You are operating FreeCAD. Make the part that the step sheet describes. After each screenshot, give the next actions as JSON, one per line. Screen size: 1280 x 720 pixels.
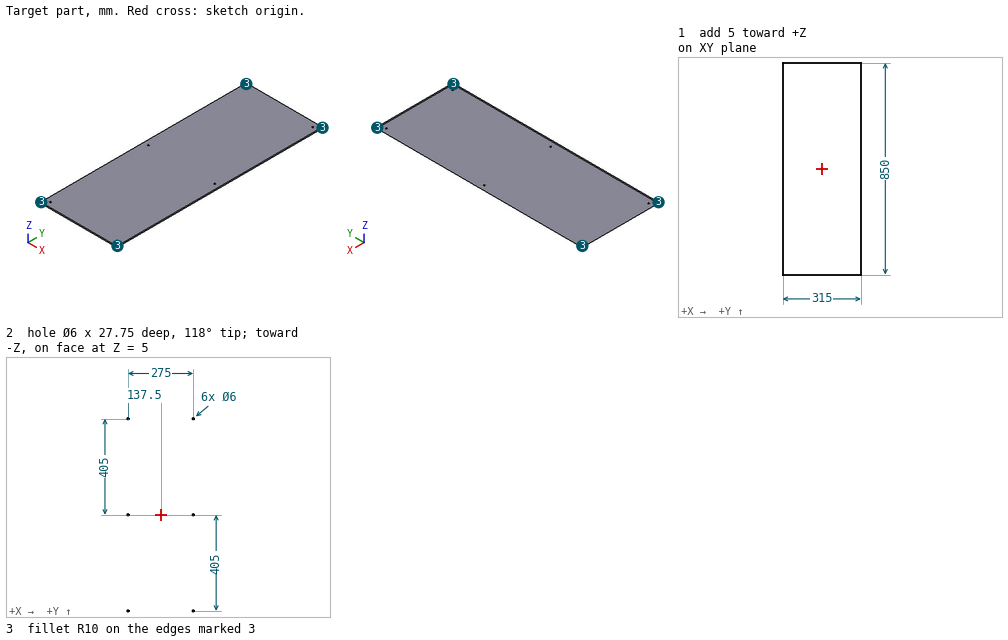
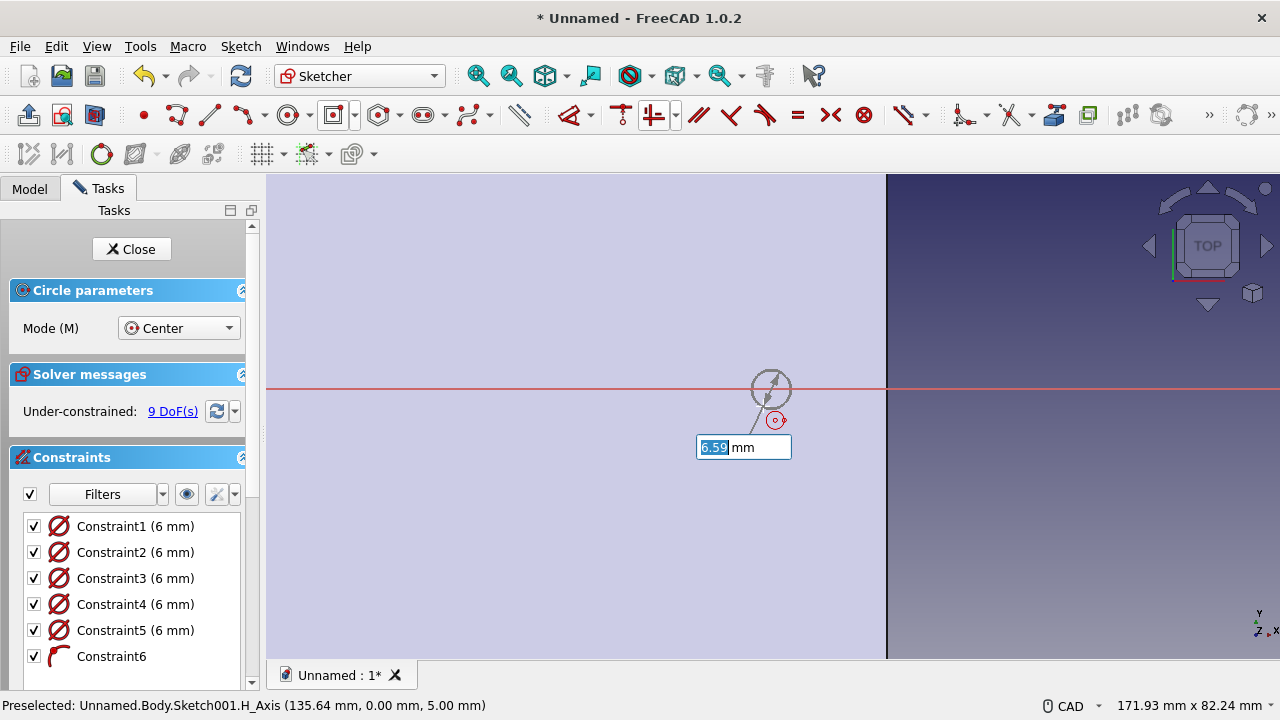
{"action": "type", "text": "6"}
{"action": "key", "text": "Return"}
{"action": "key", "text": "Escape"}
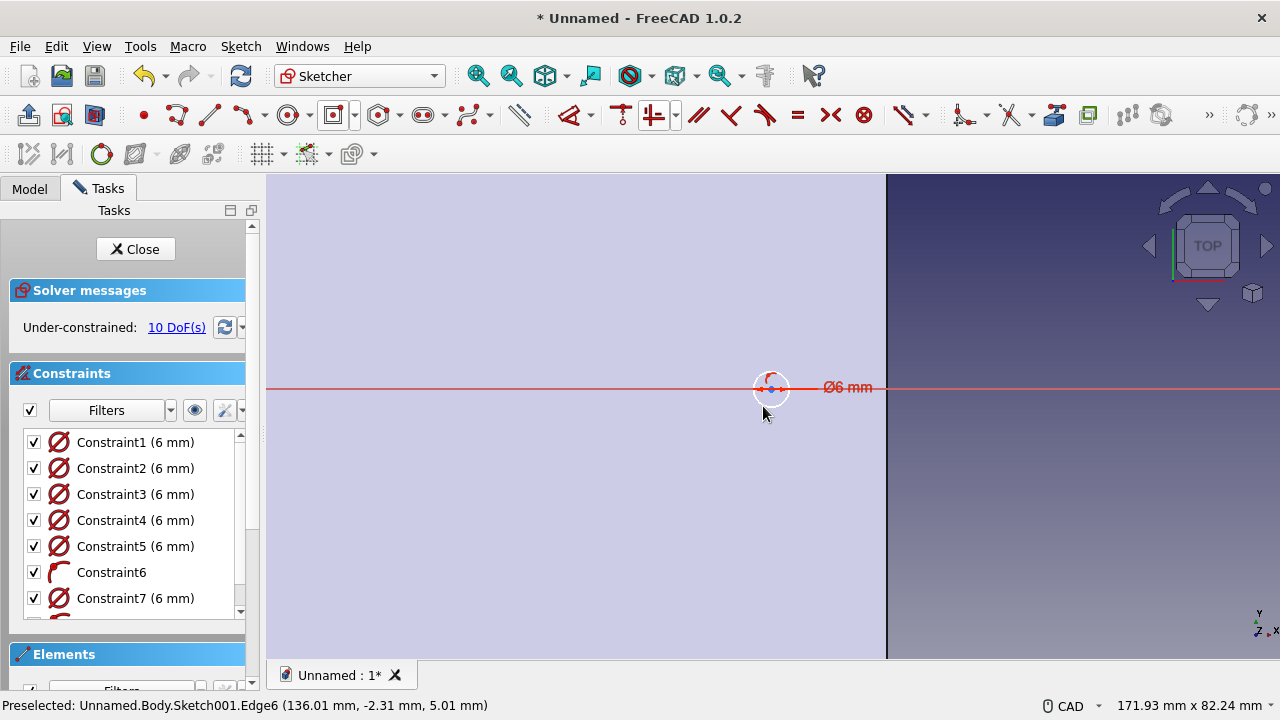
{"action": "scroll", "coordinate": [753, 418], "scroll_direction": "down", "scroll_amount": 14}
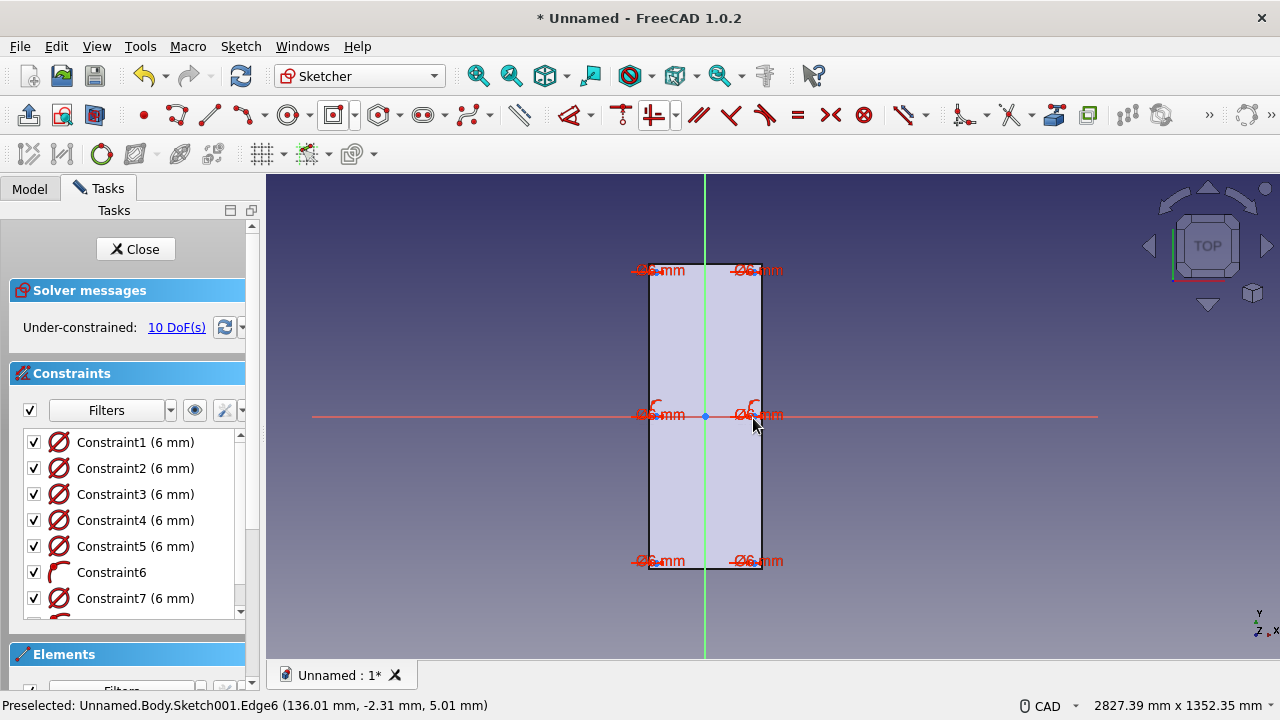
{"action": "left_click", "coordinate": [656, 272]}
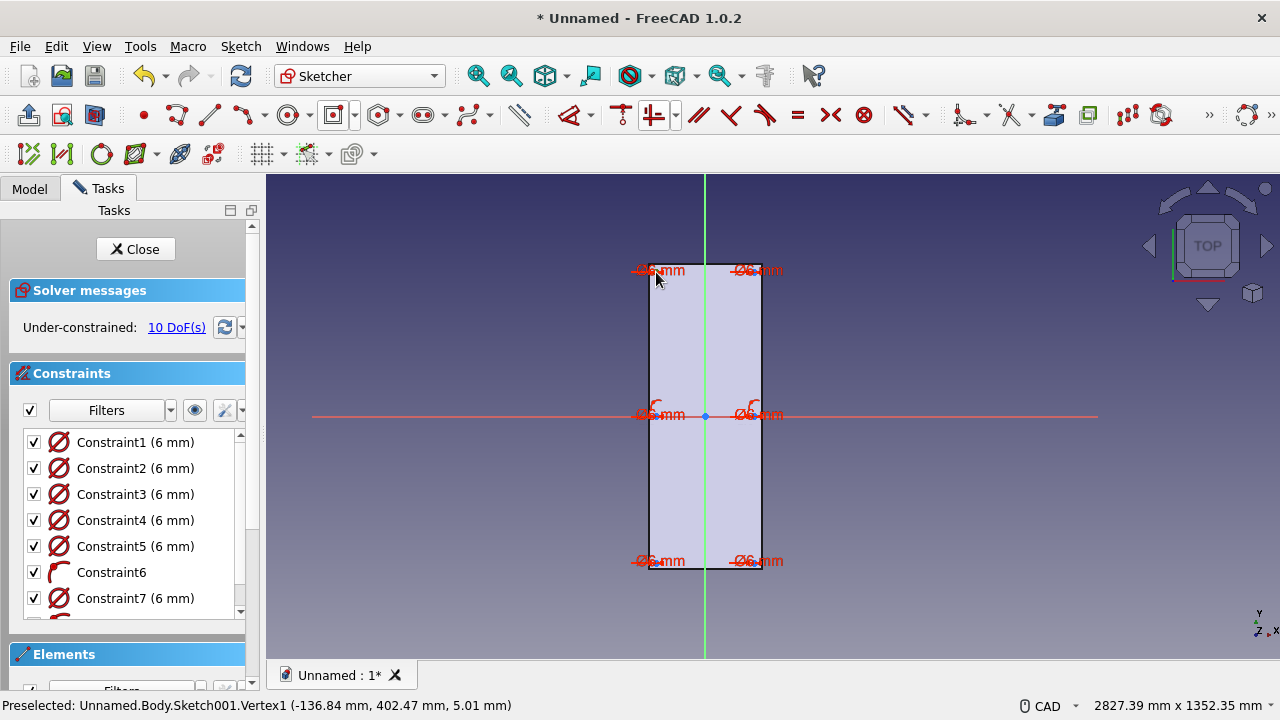
{"action": "left_click", "coordinate": [754, 272]}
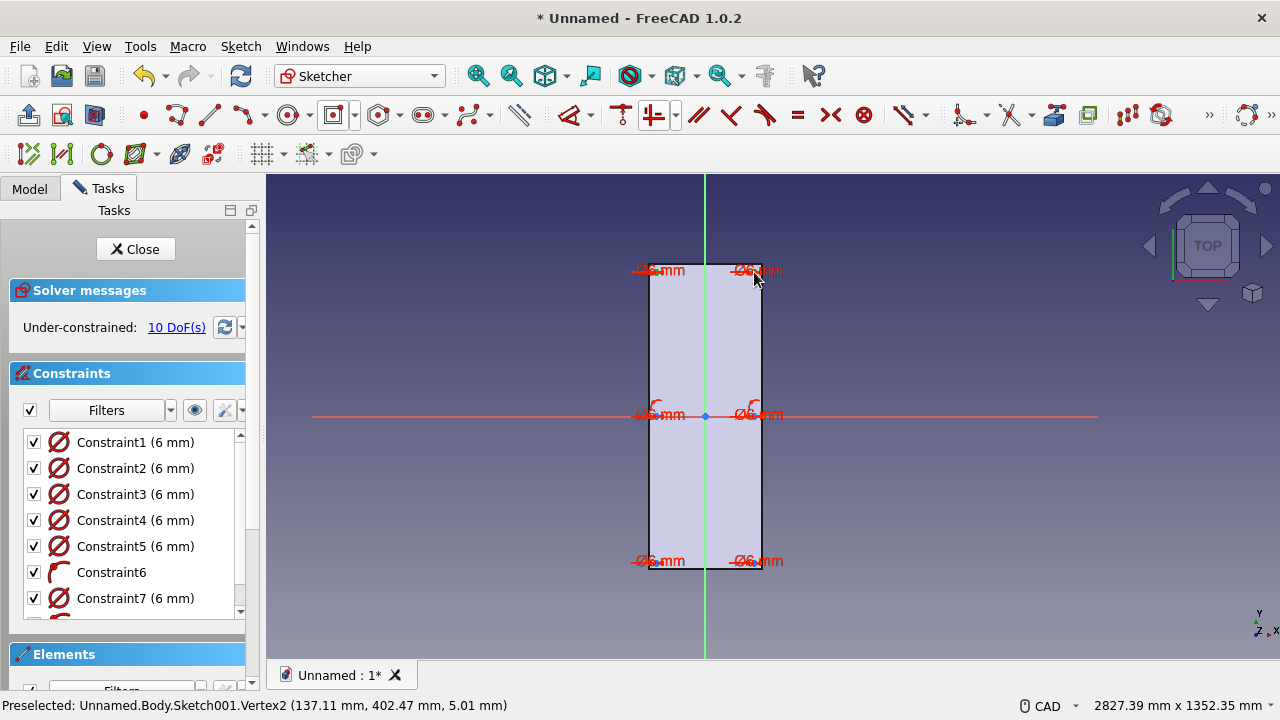
{"action": "key", "text": "h"}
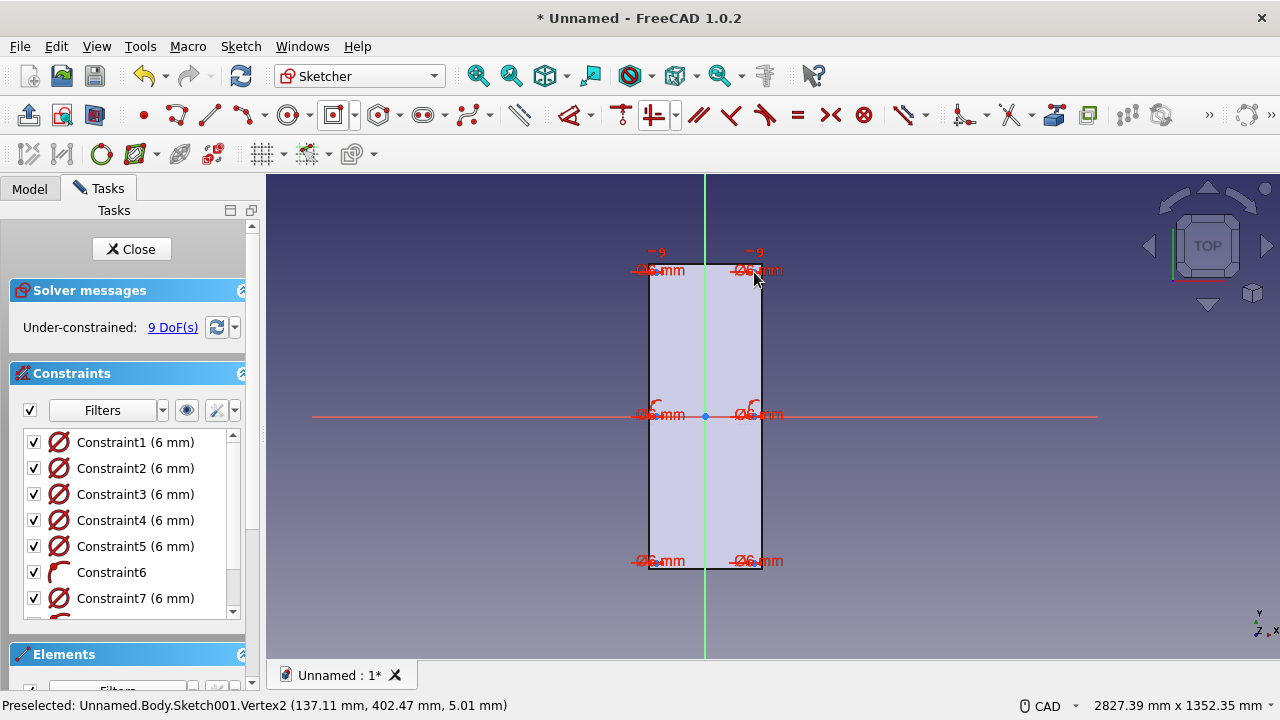
{"action": "left_click", "coordinate": [754, 272]}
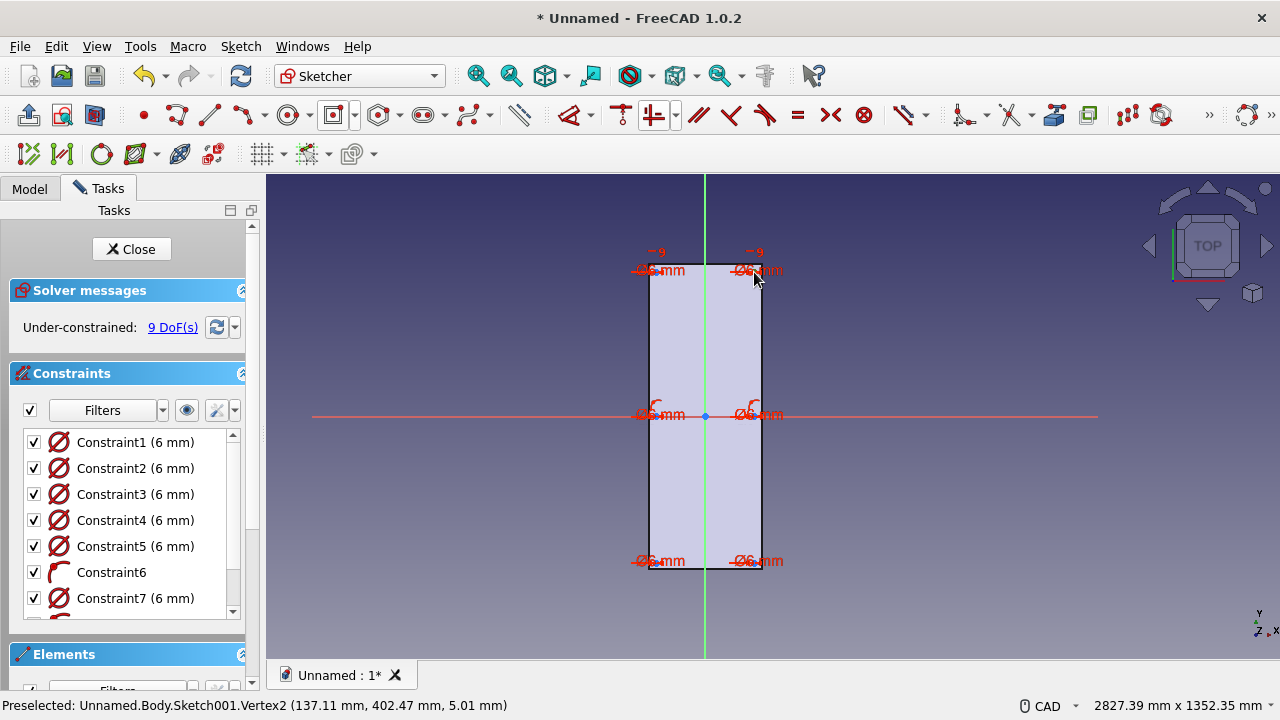
{"action": "left_click", "coordinate": [754, 563]}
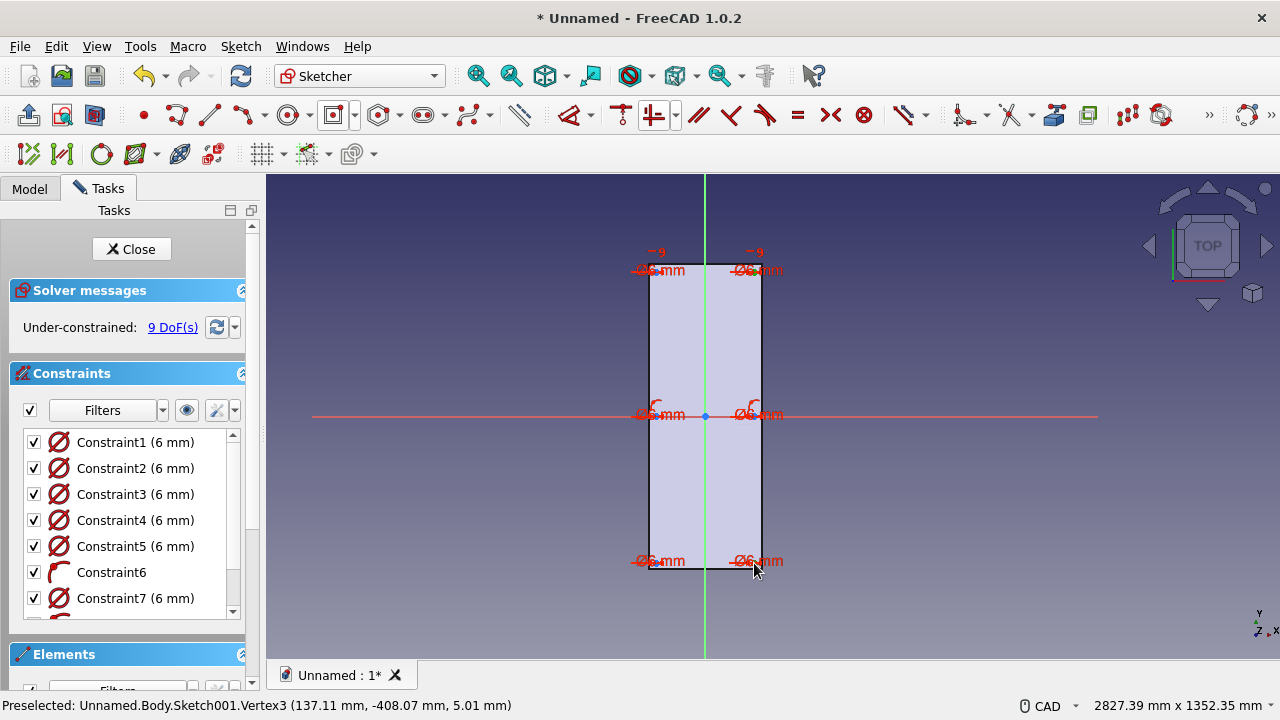
{"action": "key", "text": "v"}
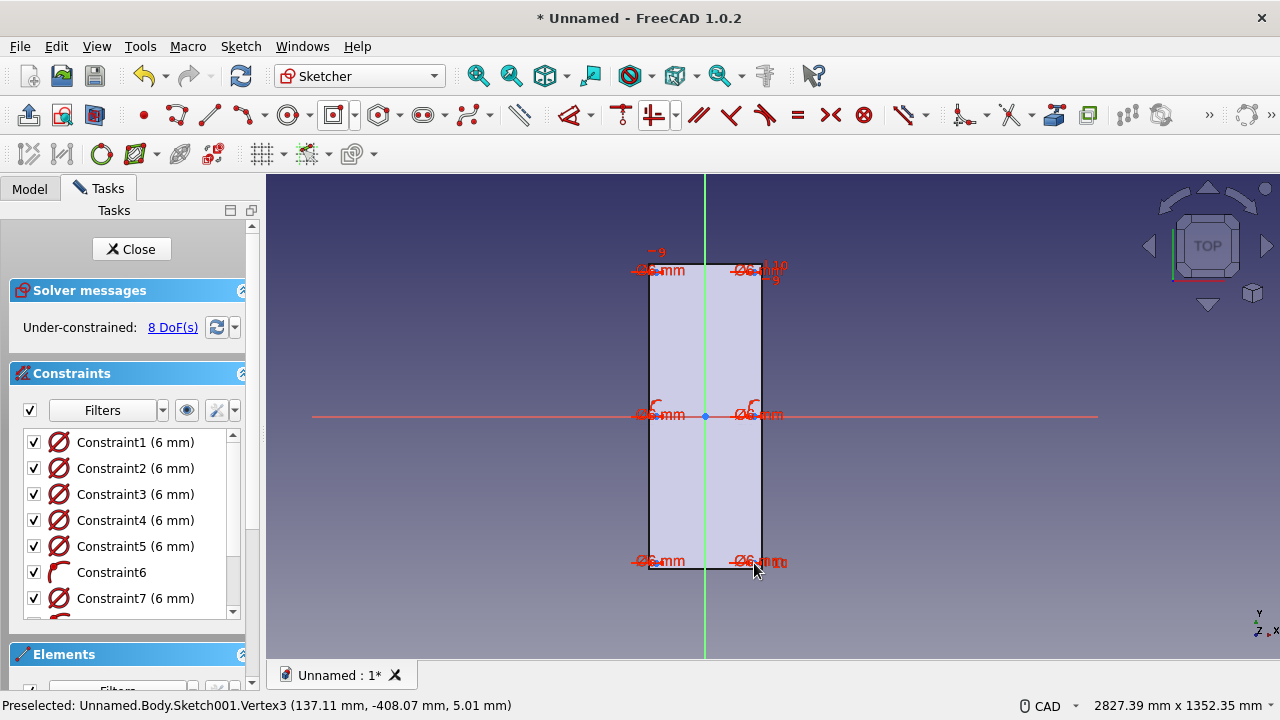
{"action": "left_click", "coordinate": [656, 272]}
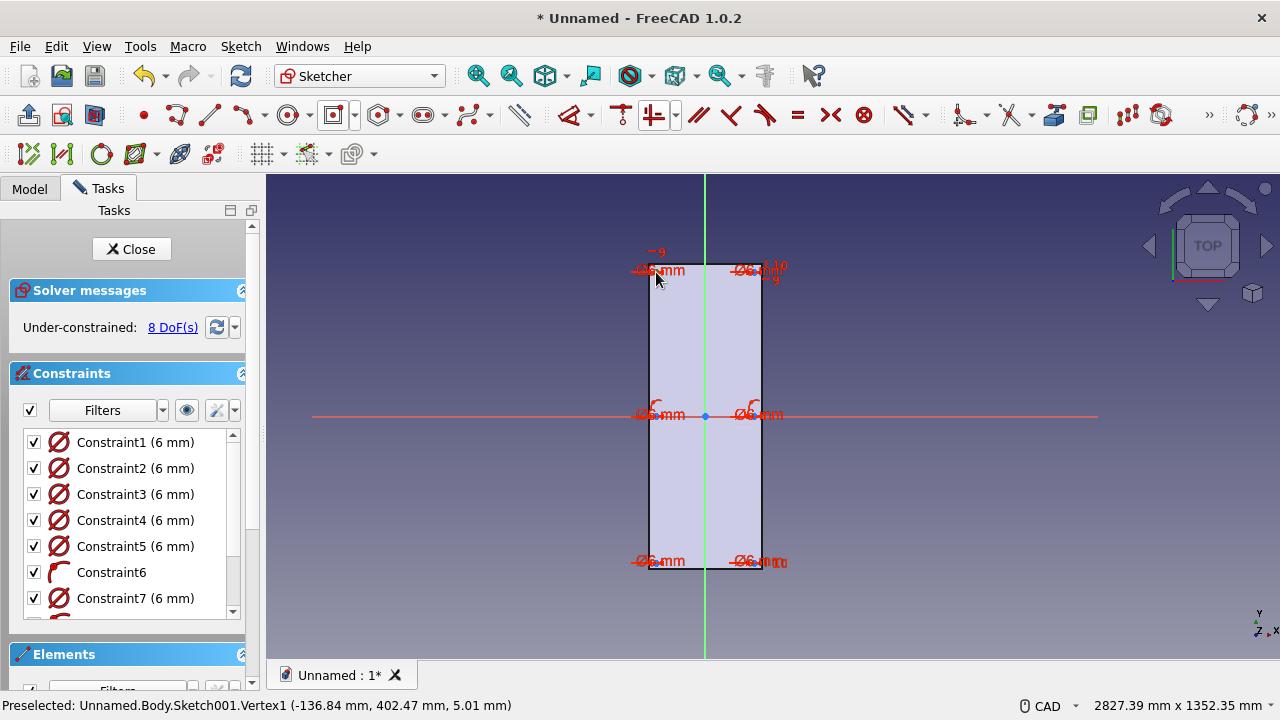
{"action": "left_click", "coordinate": [656, 563]}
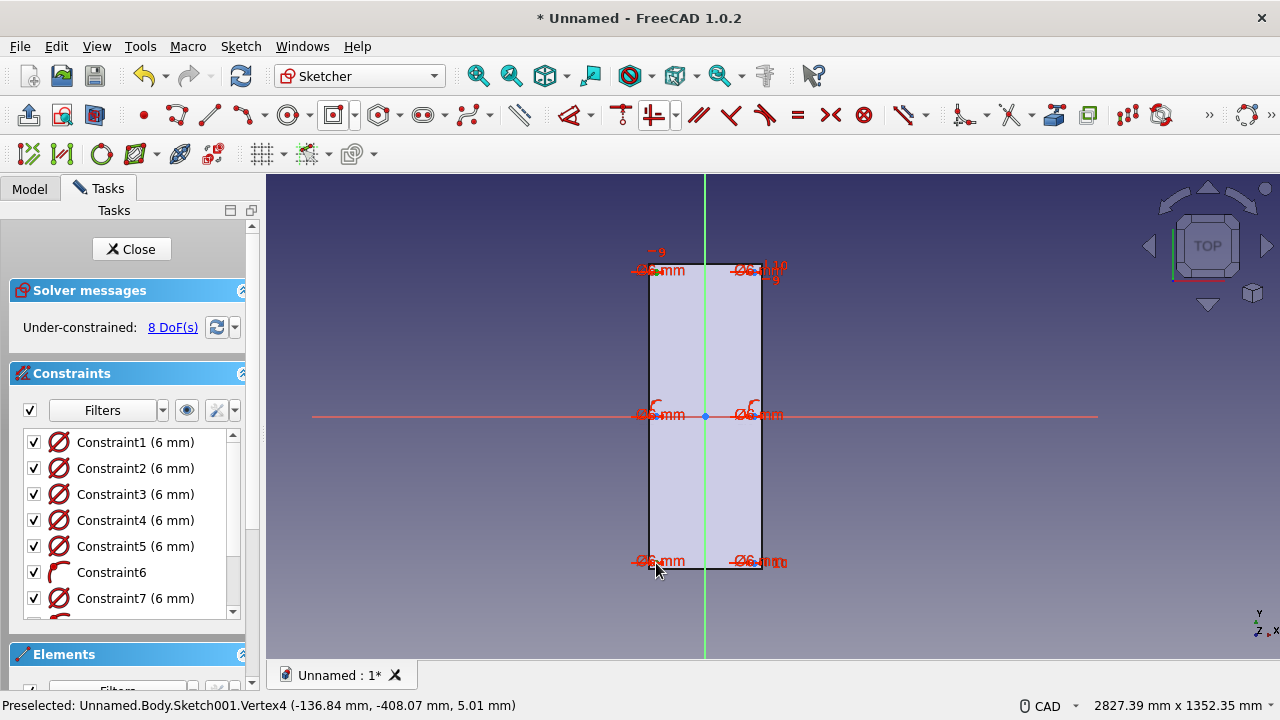
{"action": "key", "text": "v"}